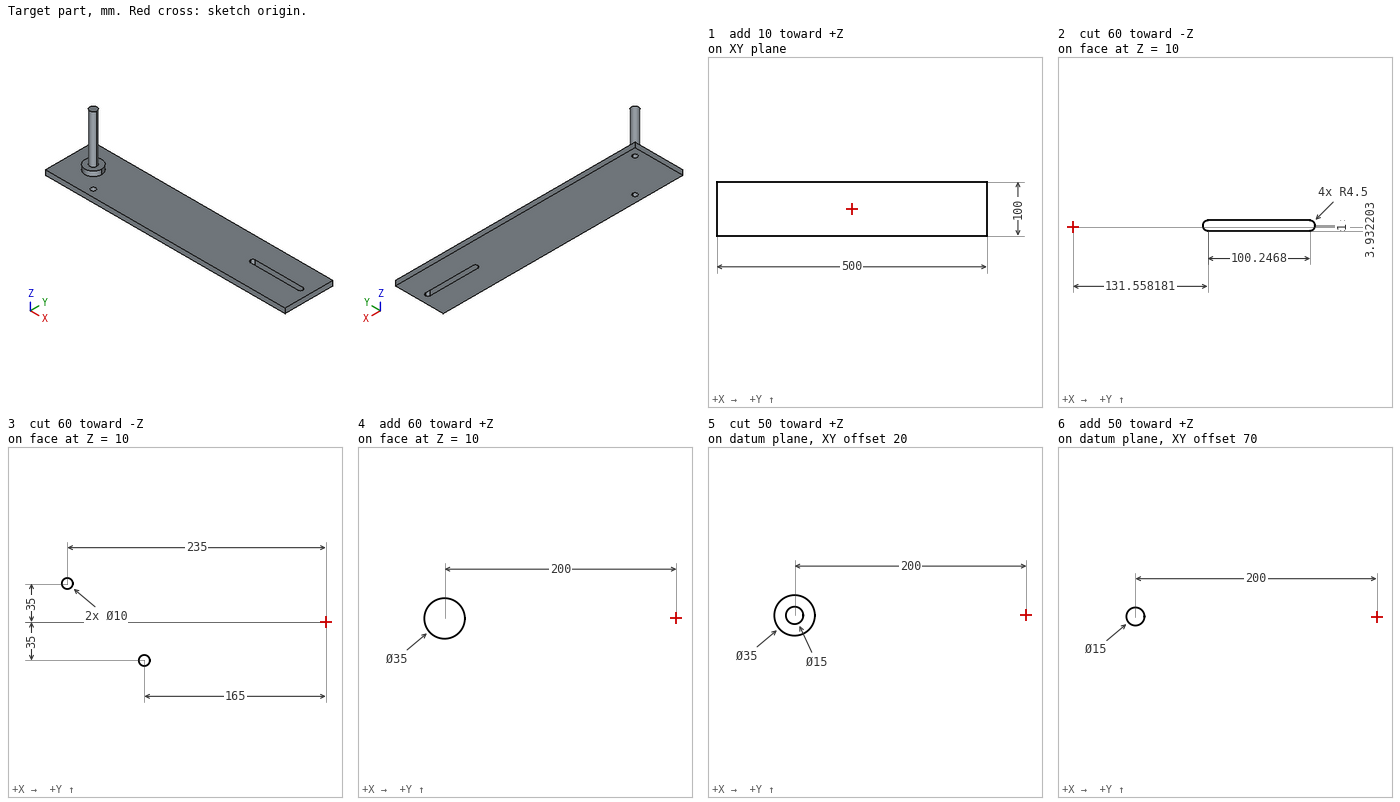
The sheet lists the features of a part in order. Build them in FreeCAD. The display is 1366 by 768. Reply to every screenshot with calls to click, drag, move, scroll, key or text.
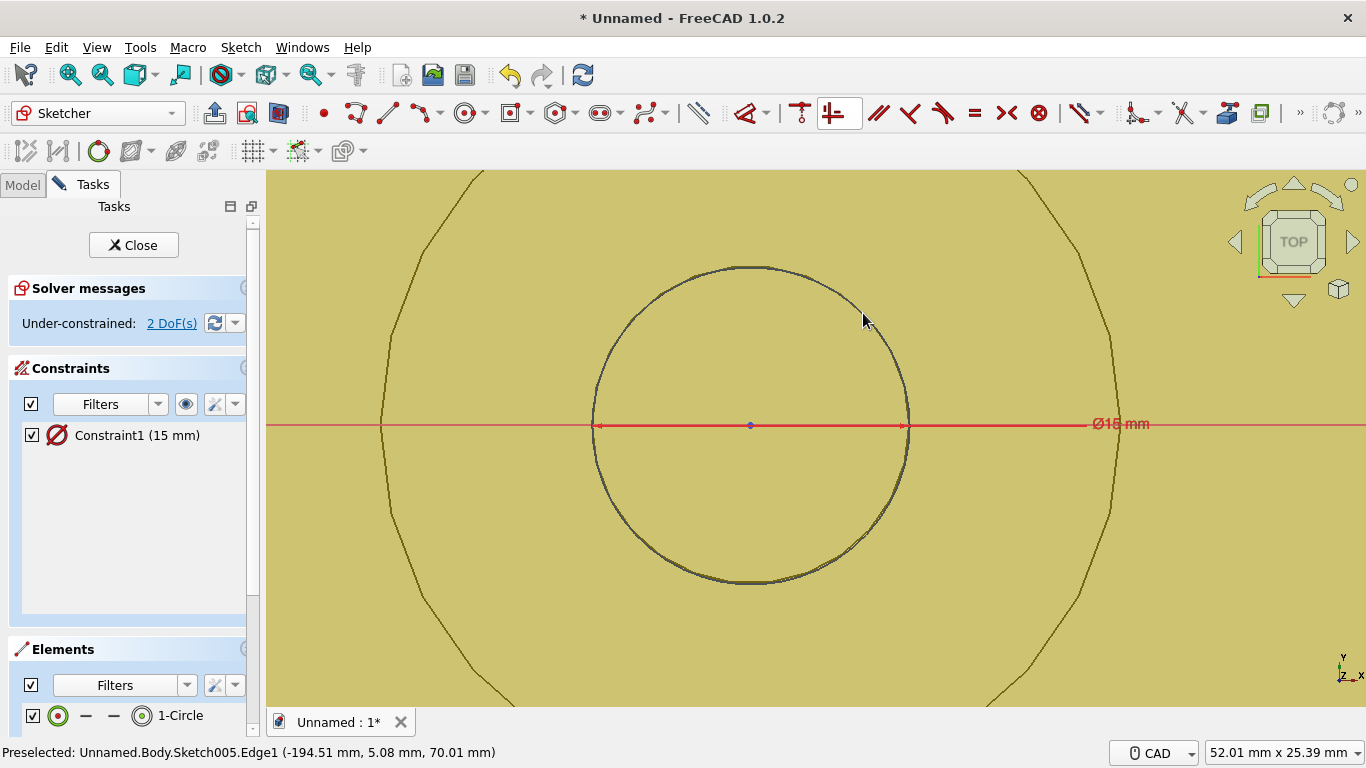
click(751, 426)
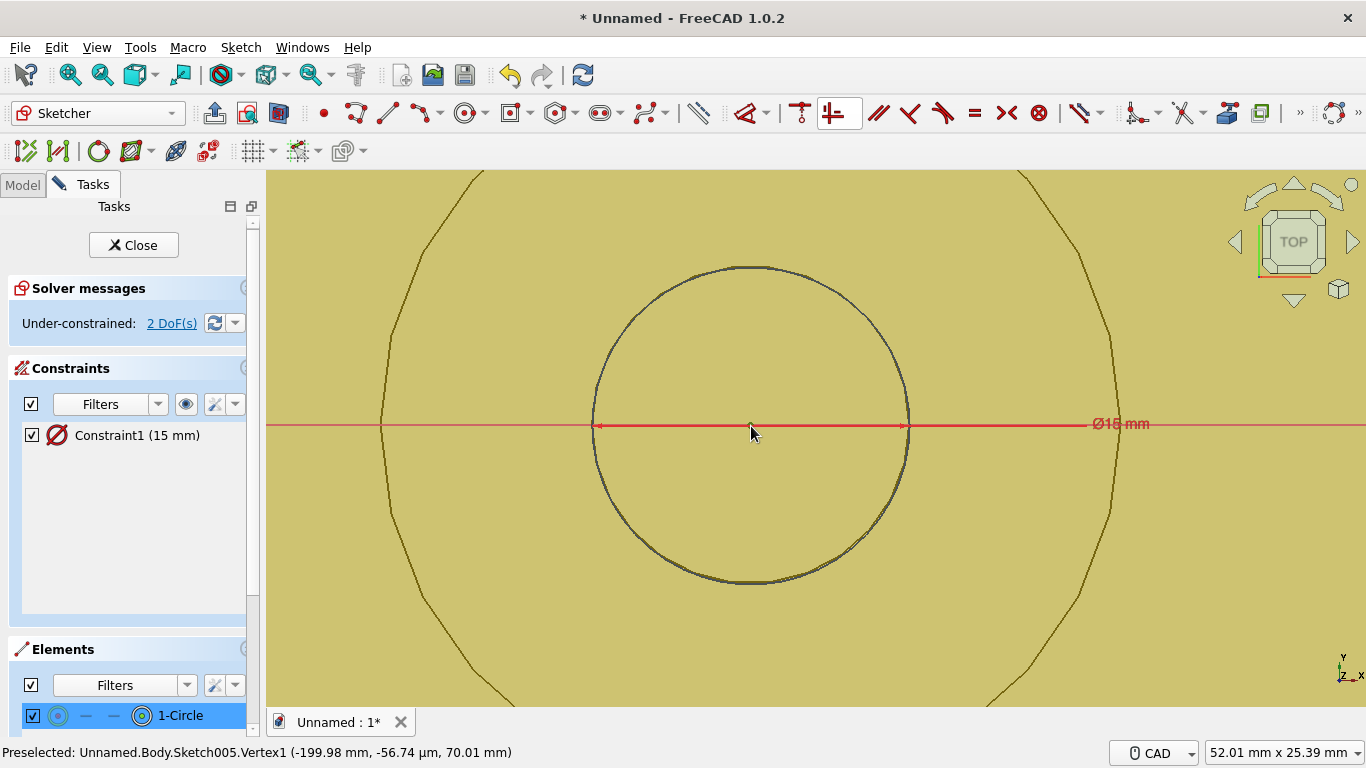
click(359, 425)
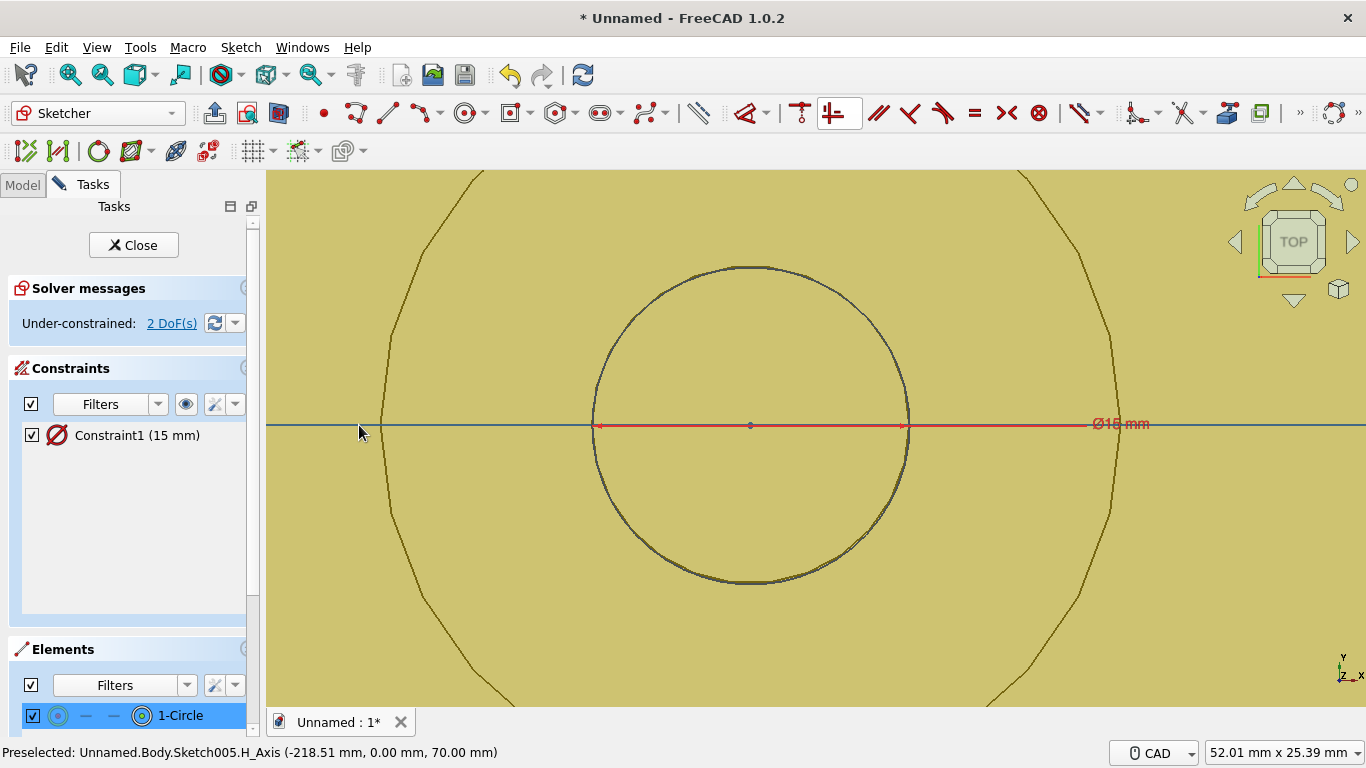
key(c)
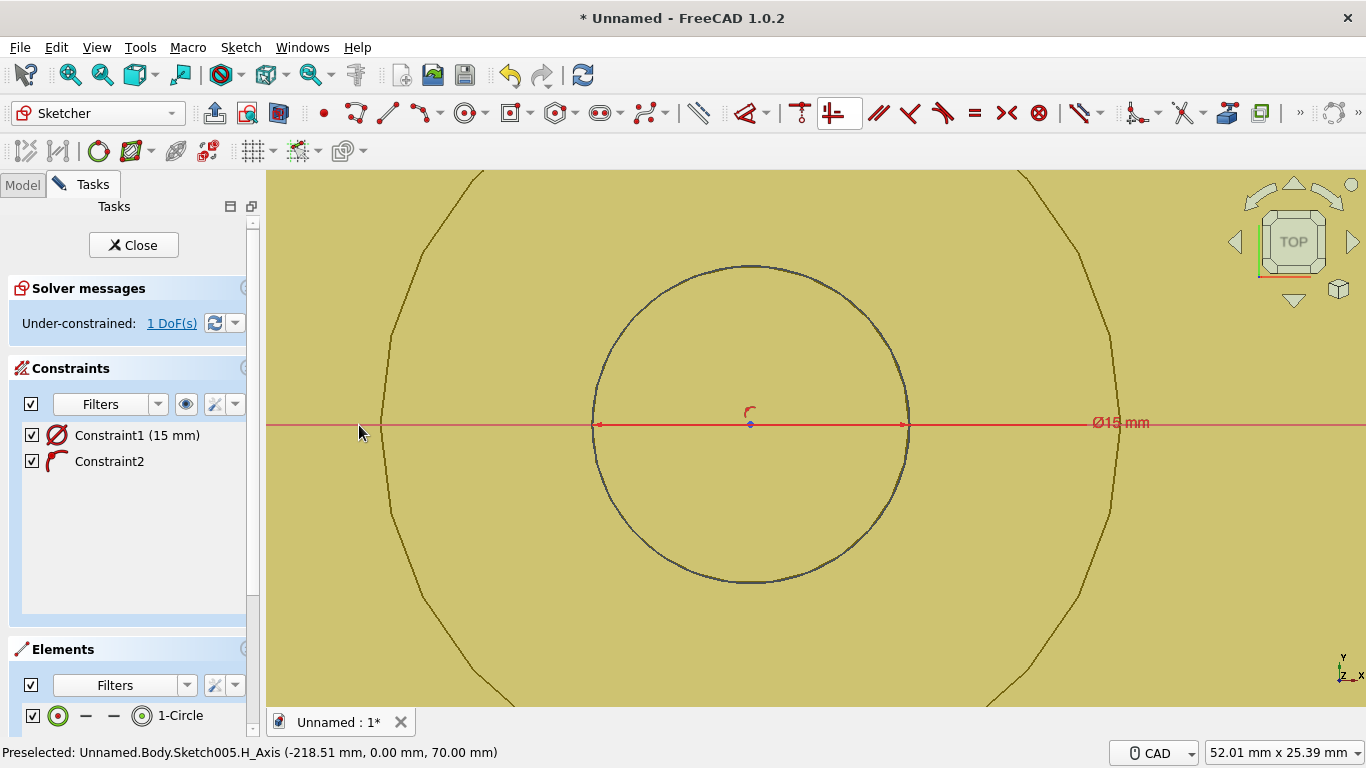
key(d)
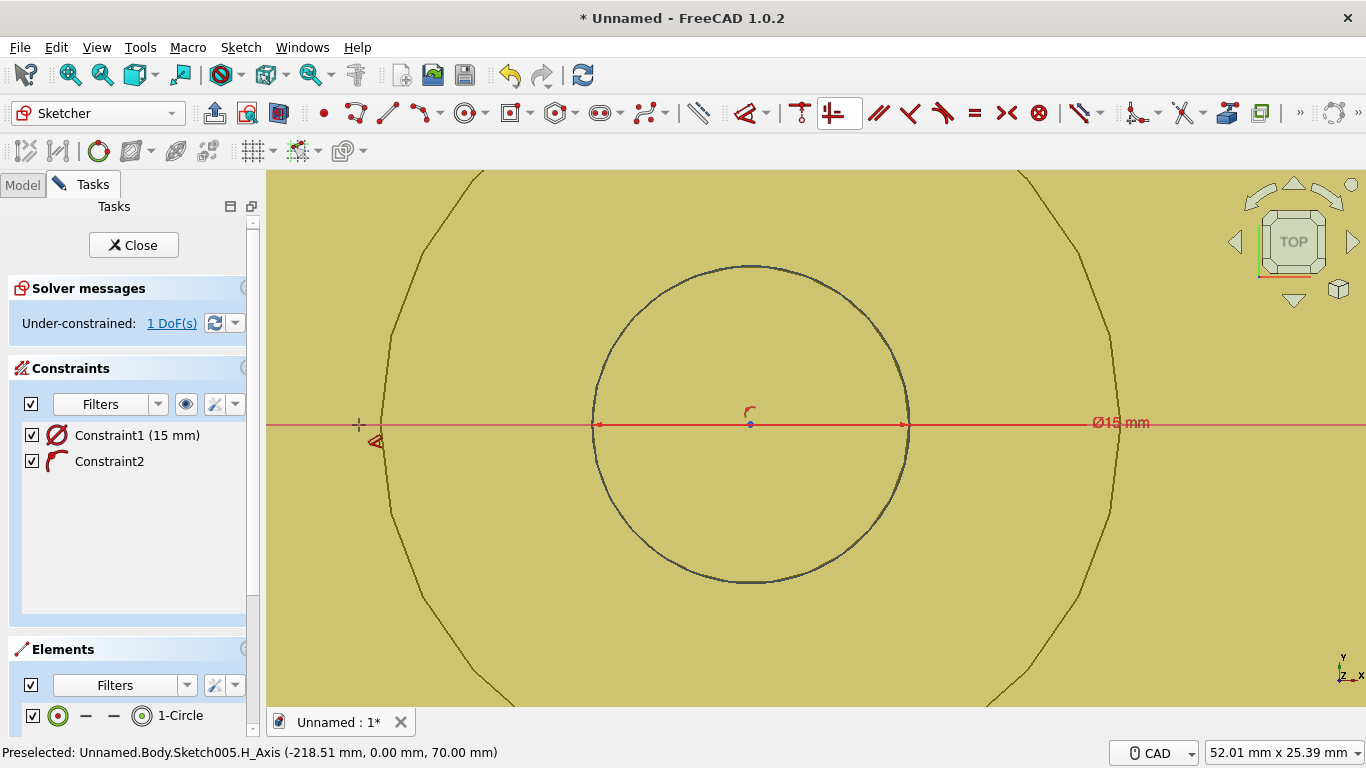
click(751, 425)
click(976, 459)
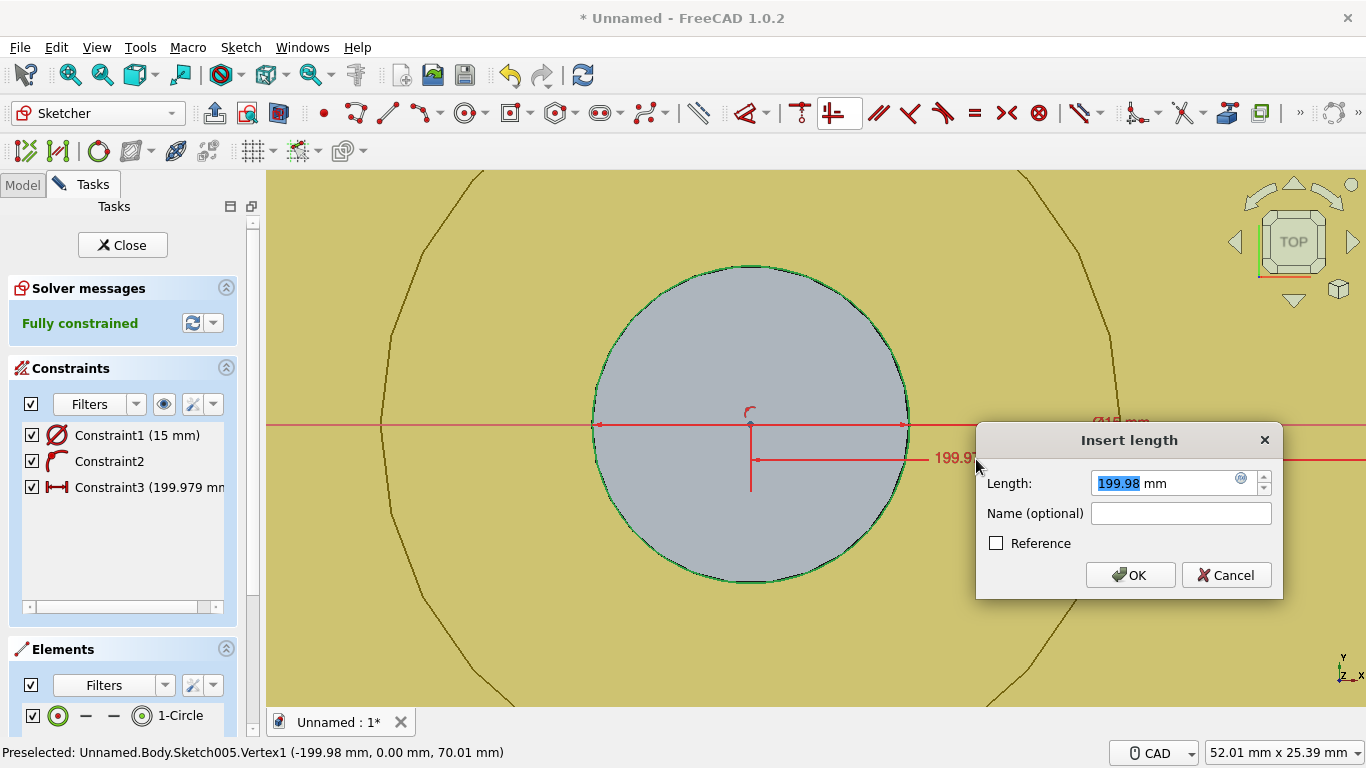
text(200)
key(Return)
key(Escape)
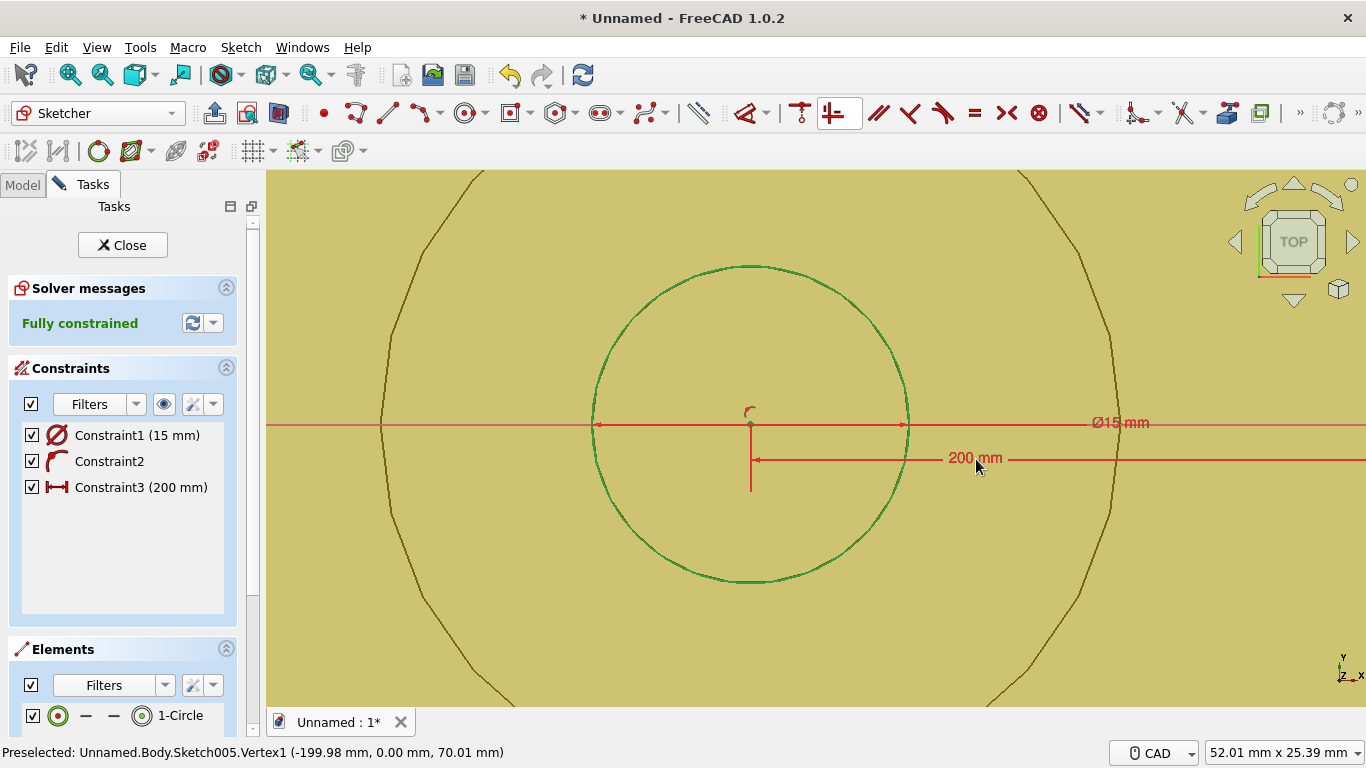
click(123, 245)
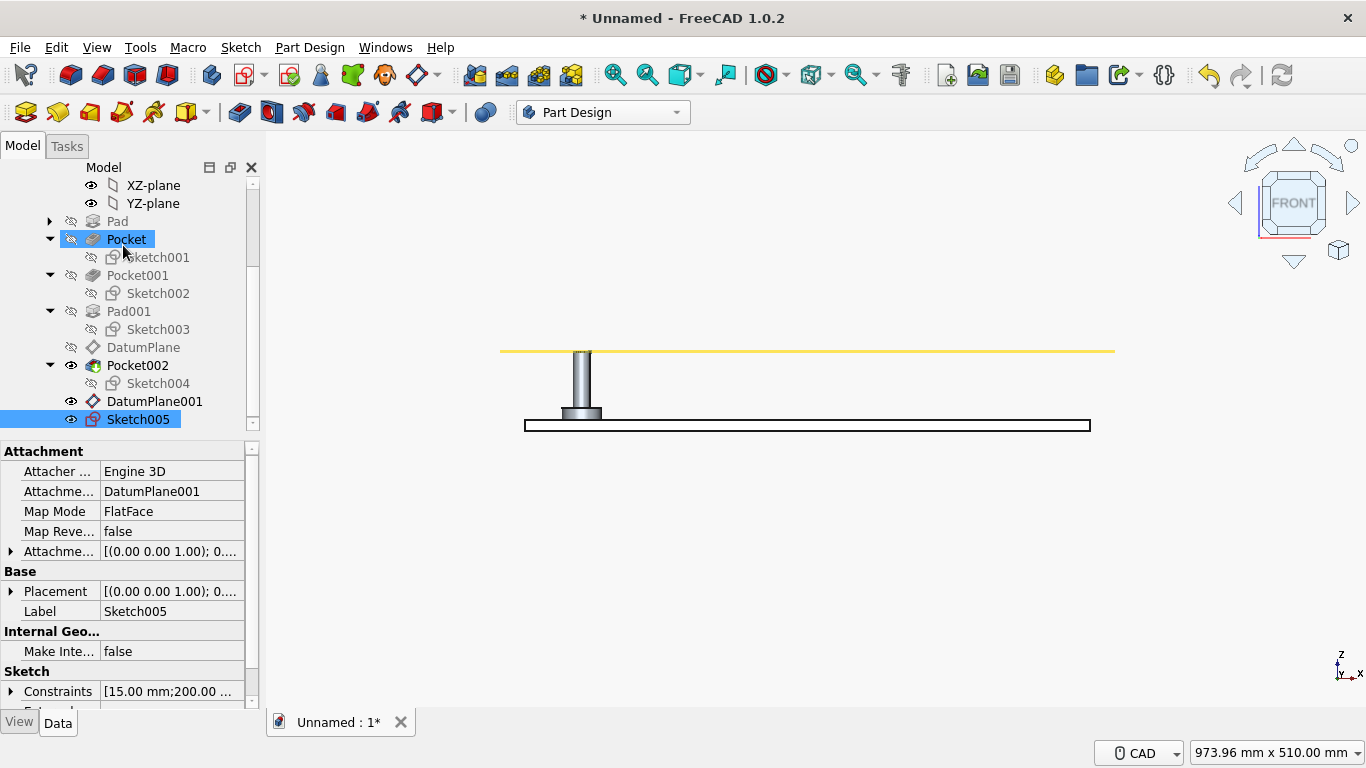
click(26, 112)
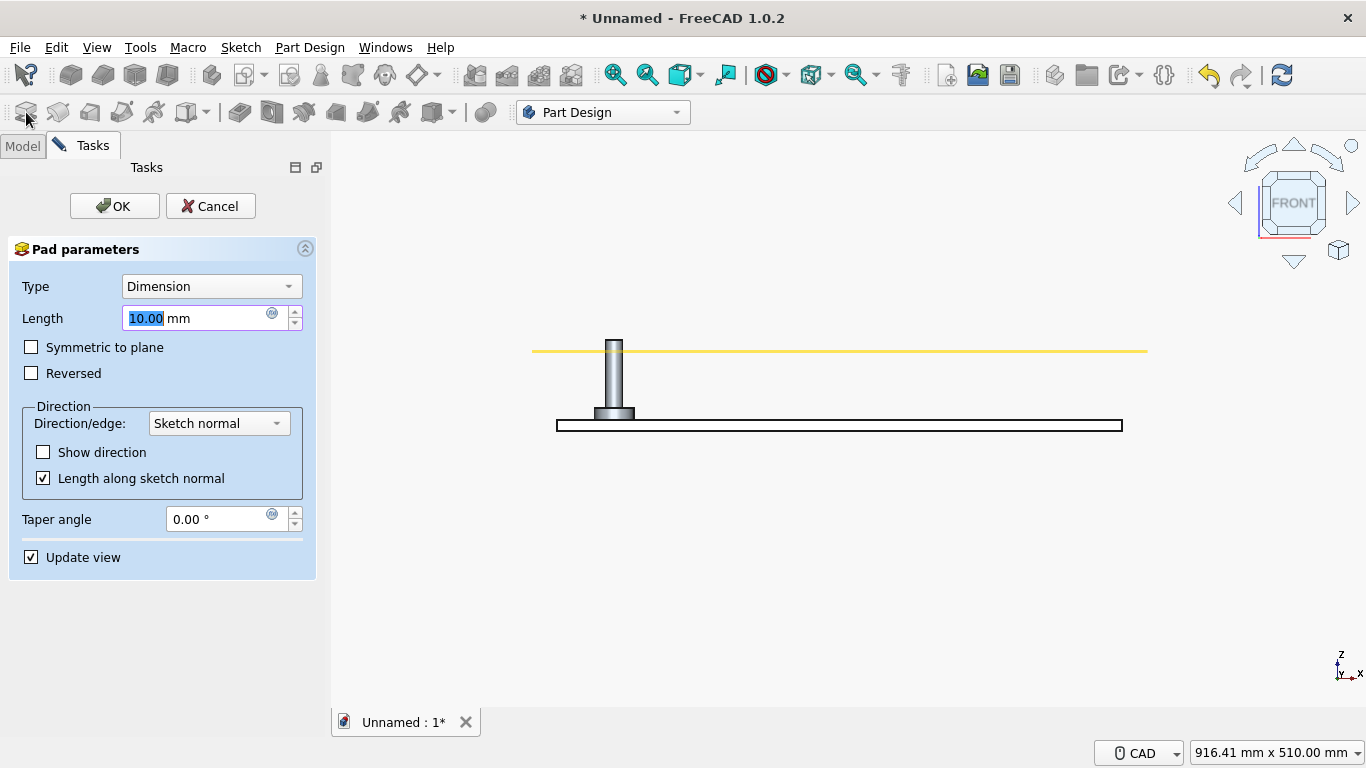
text(50)
key(Tab)